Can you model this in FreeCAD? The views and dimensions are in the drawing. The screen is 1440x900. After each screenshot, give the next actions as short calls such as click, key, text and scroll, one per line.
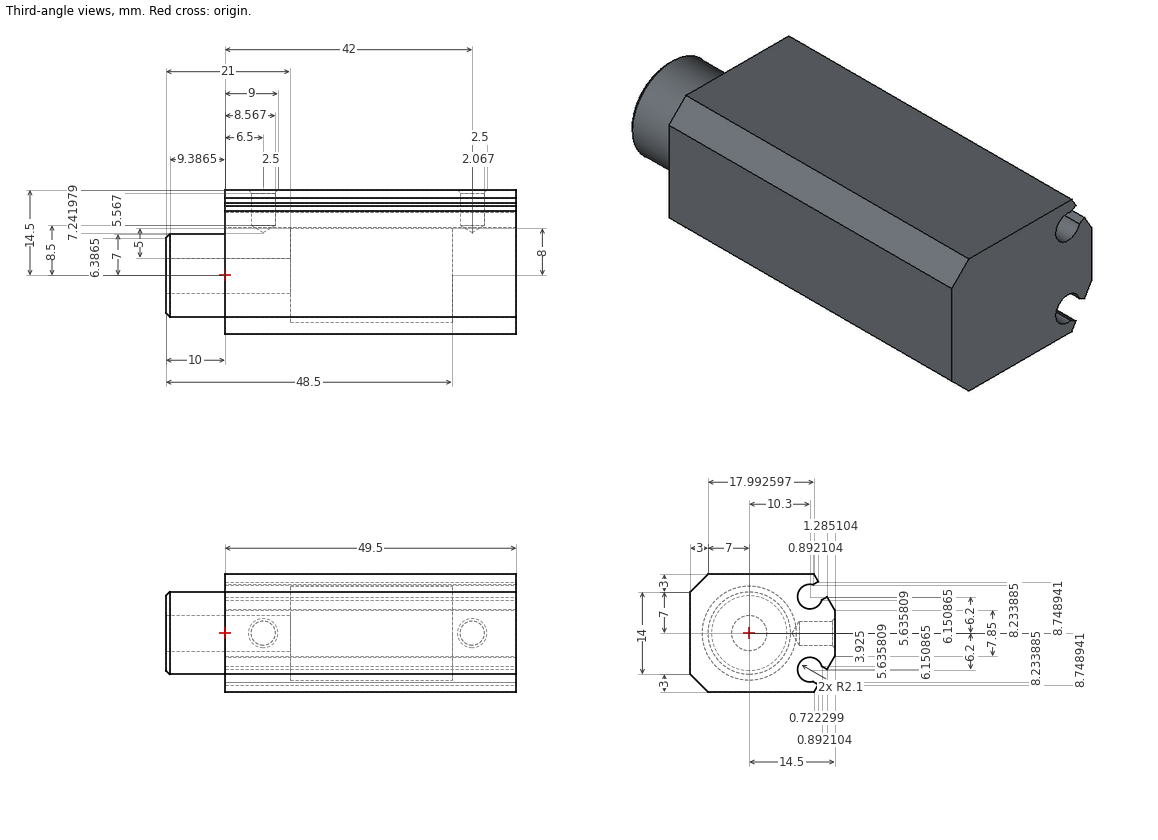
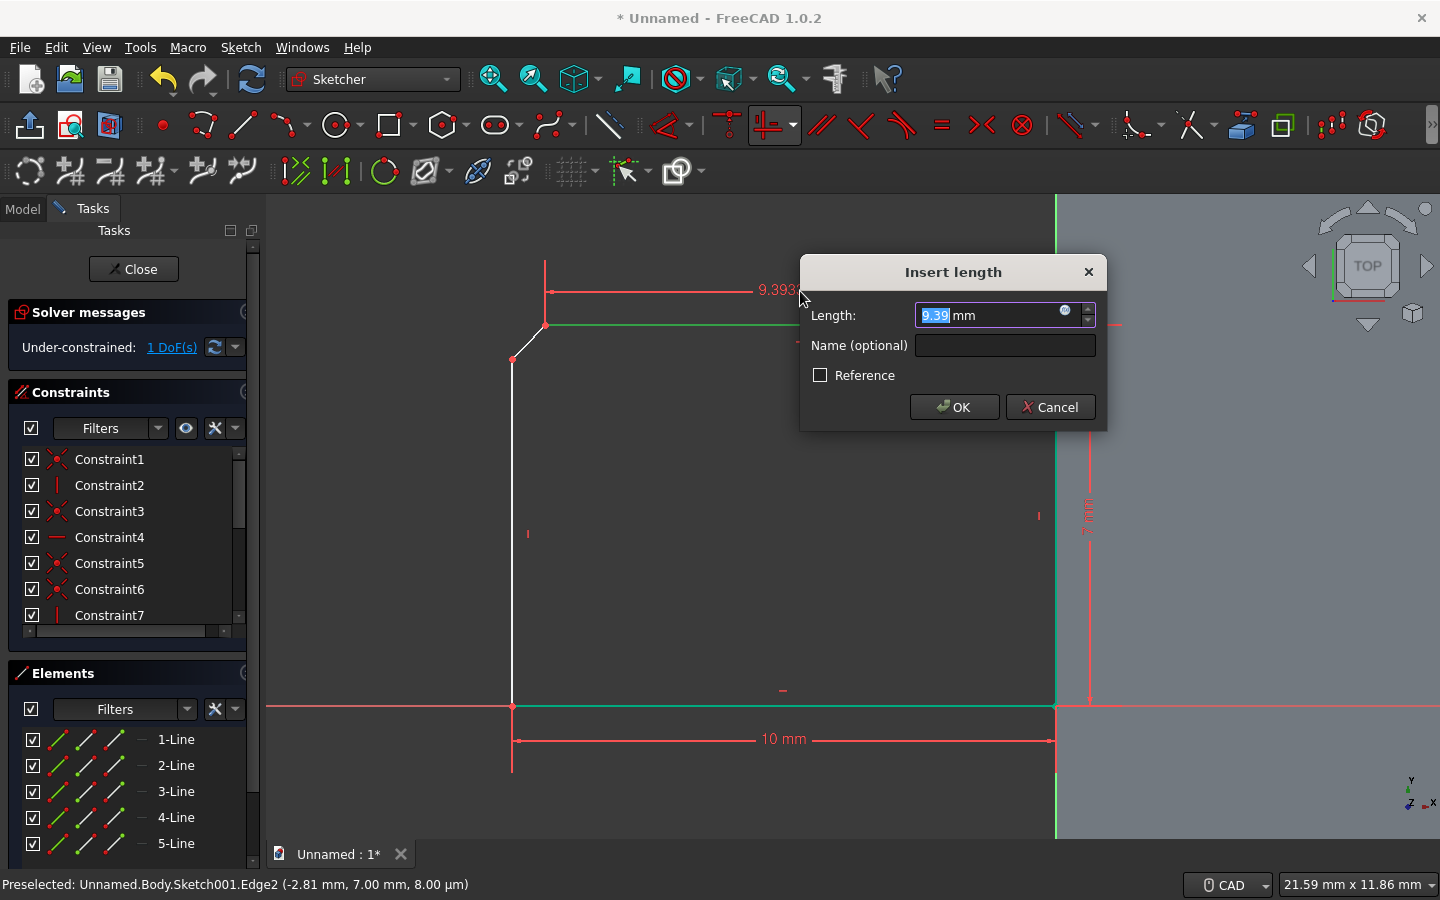
text(9.3865)
key(Return)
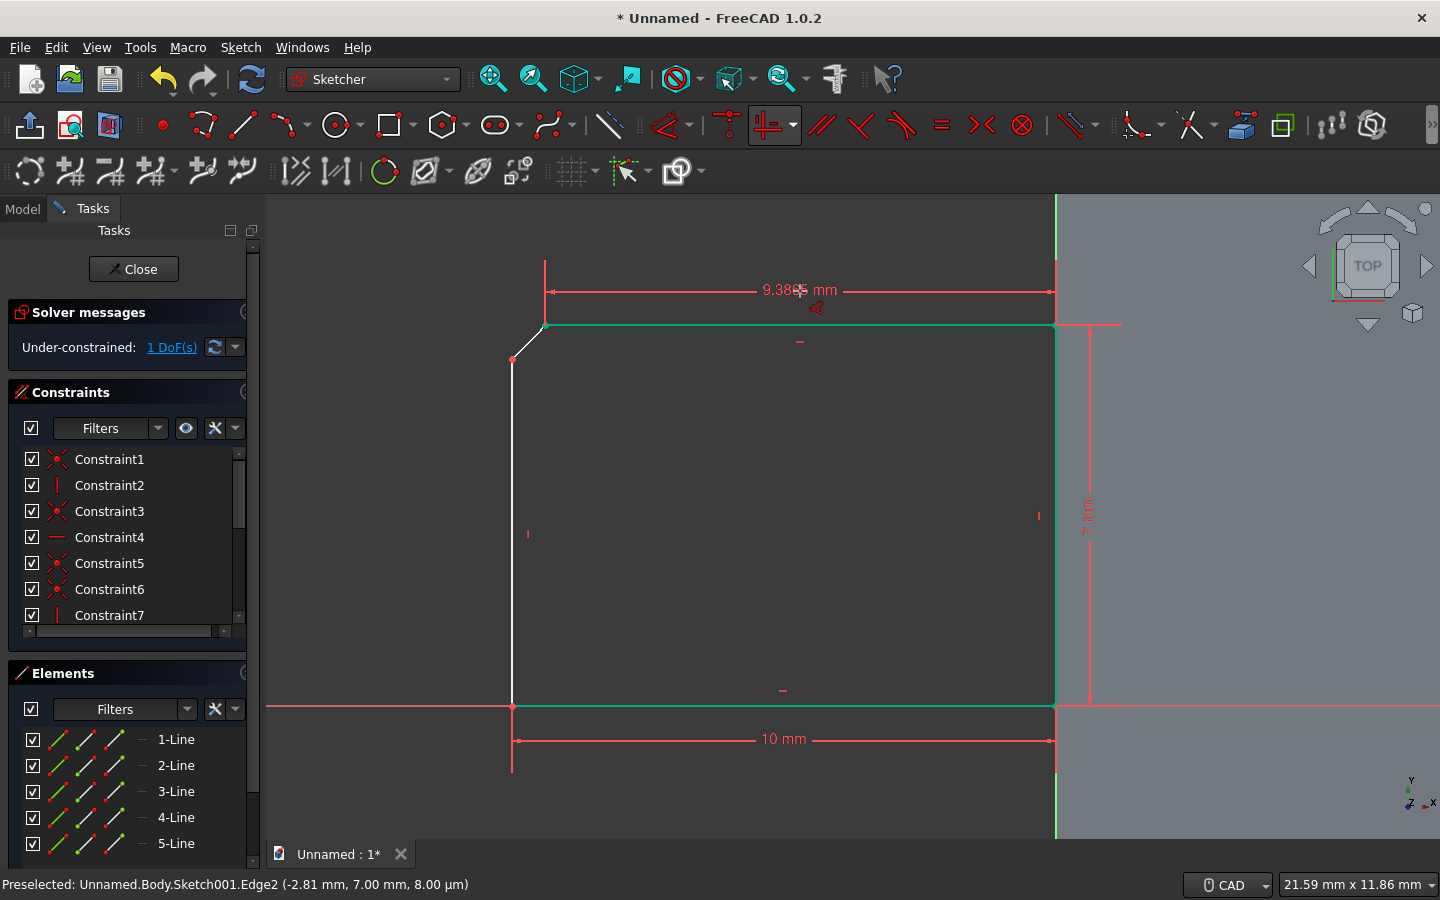
click(512, 464)
click(478, 533)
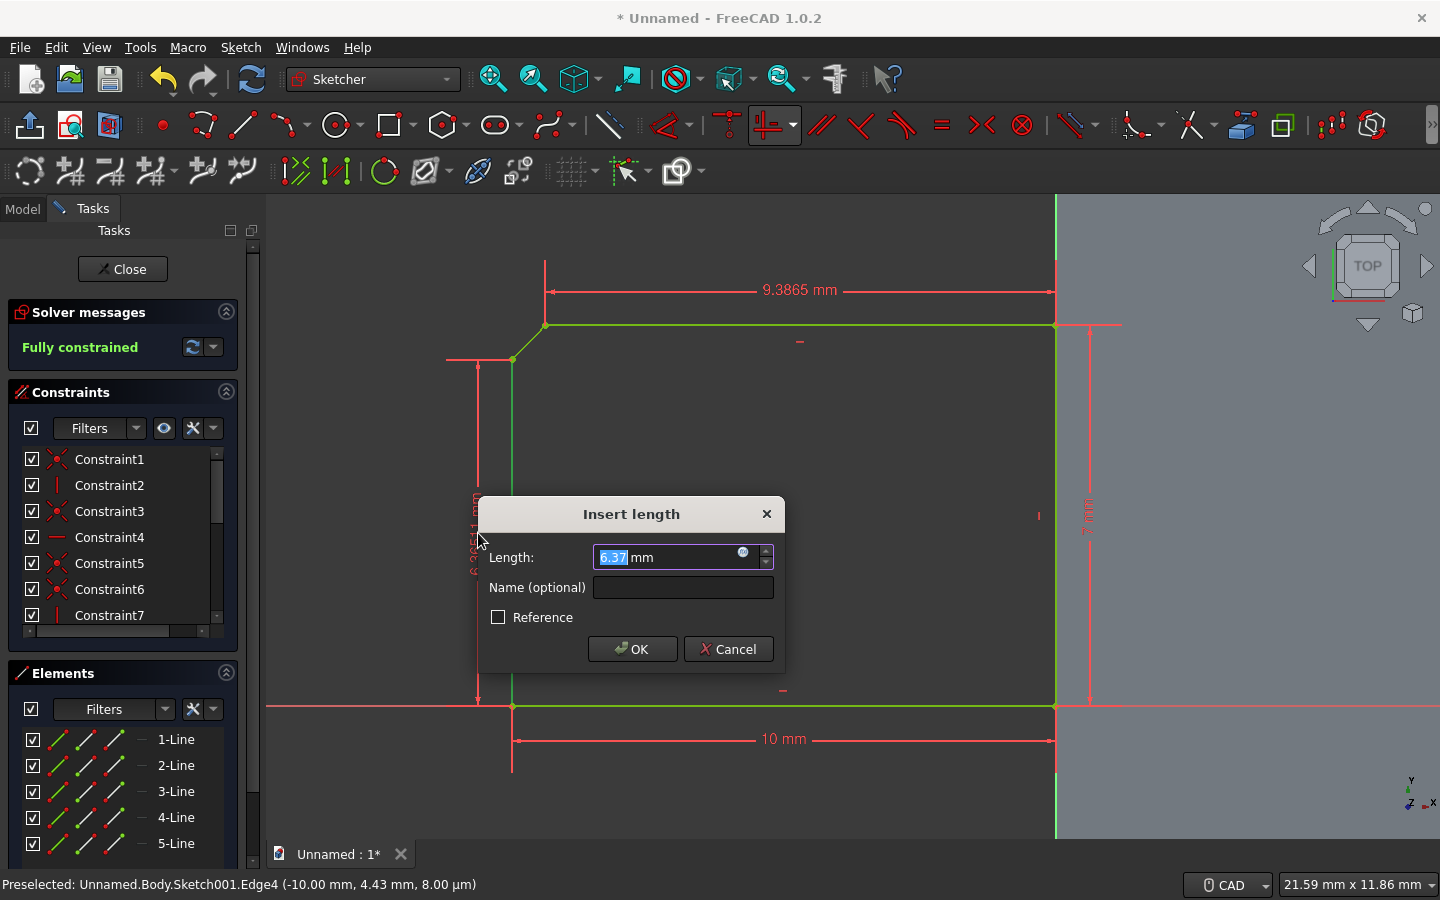
text(6.3865)
key(Return)
key(Escape)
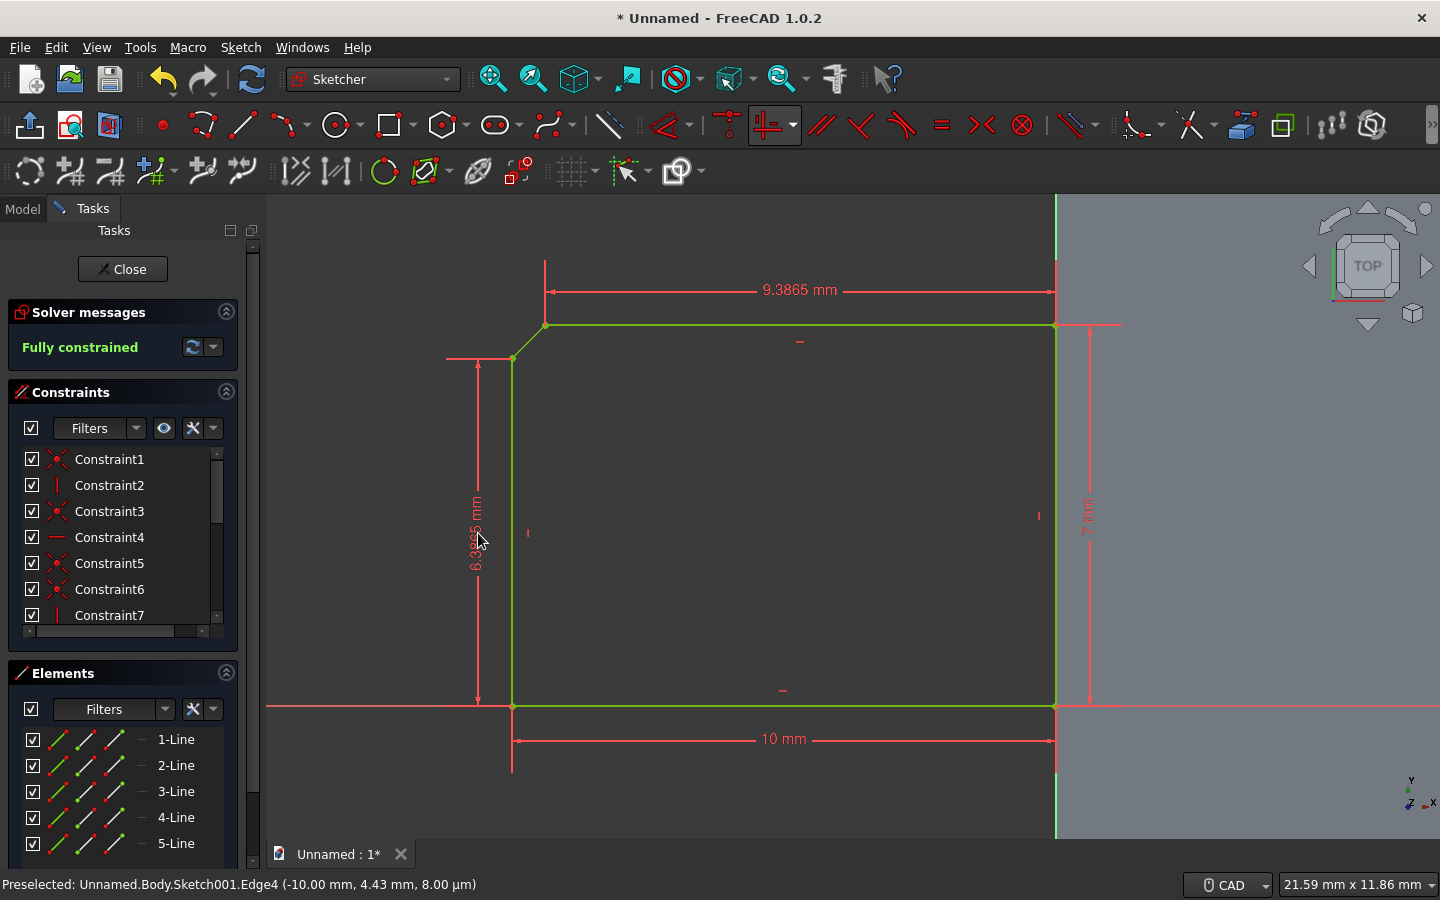
click(123, 269)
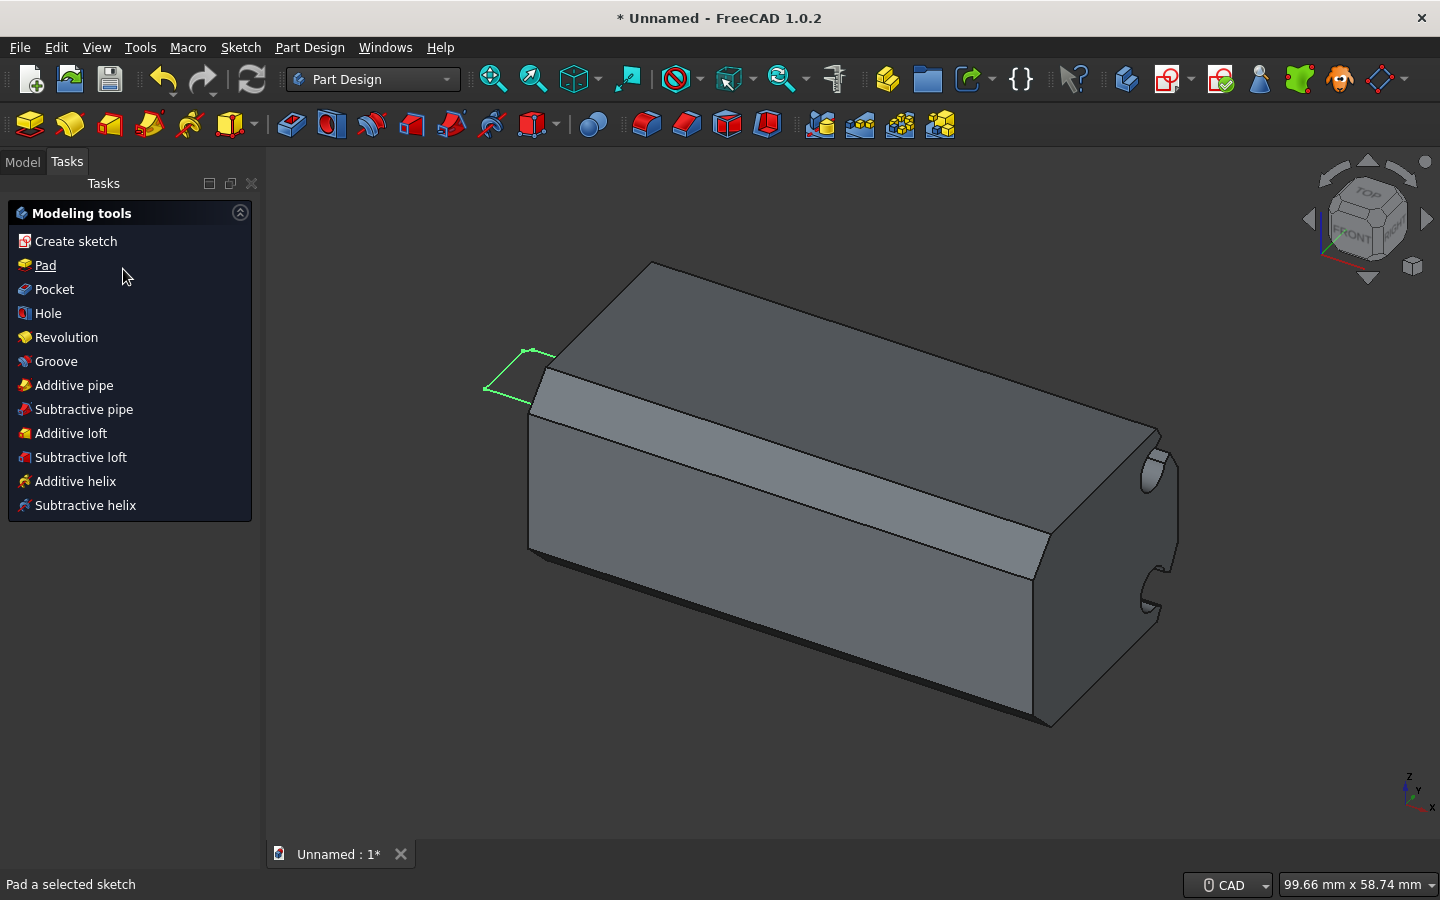
click(70, 124)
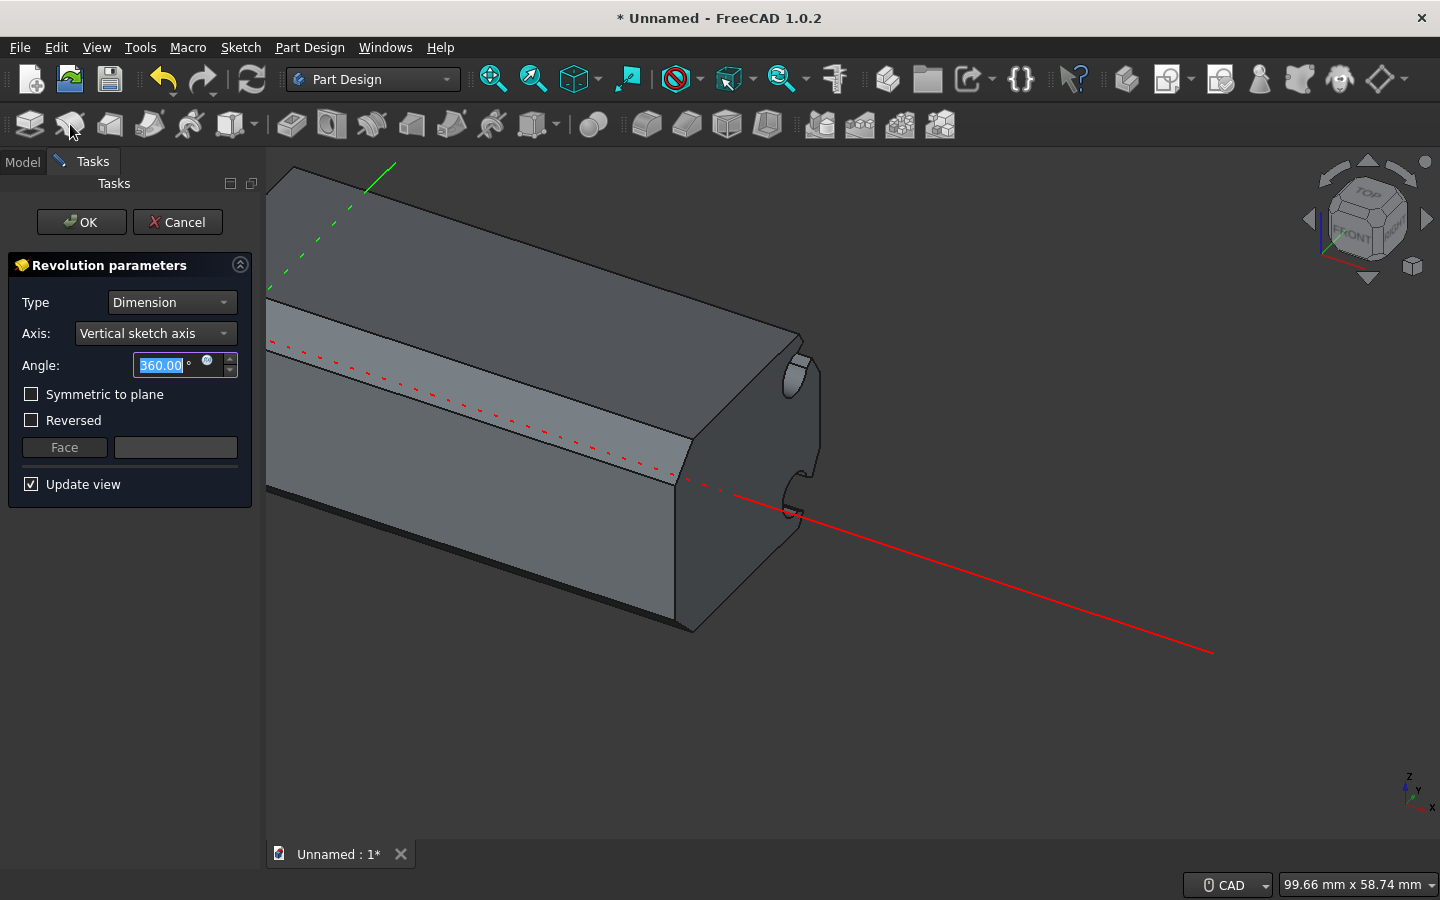
click(156, 334)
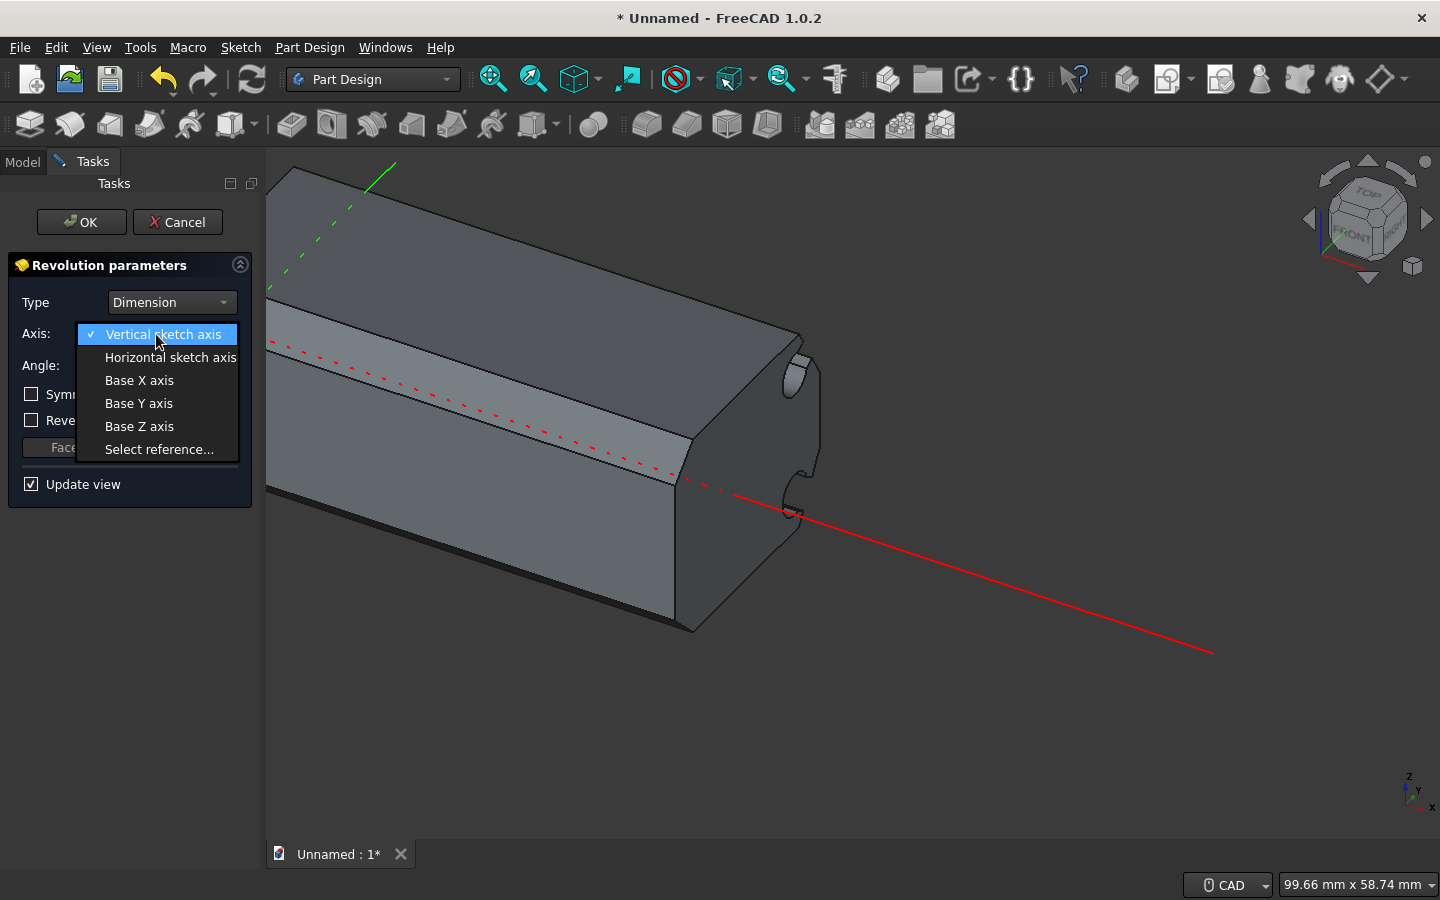
click(156, 358)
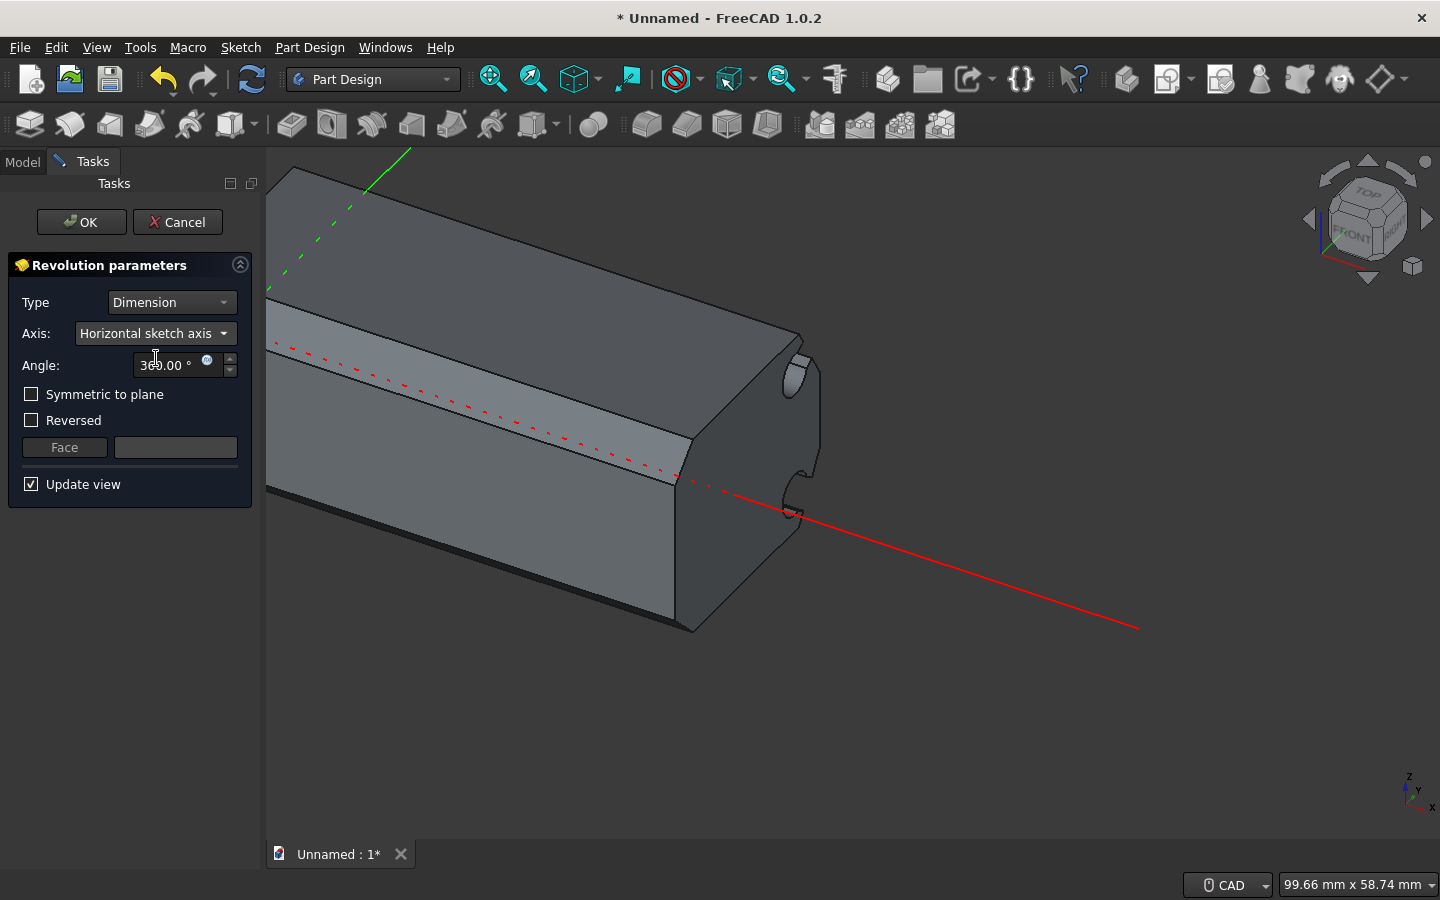
click(82, 222)